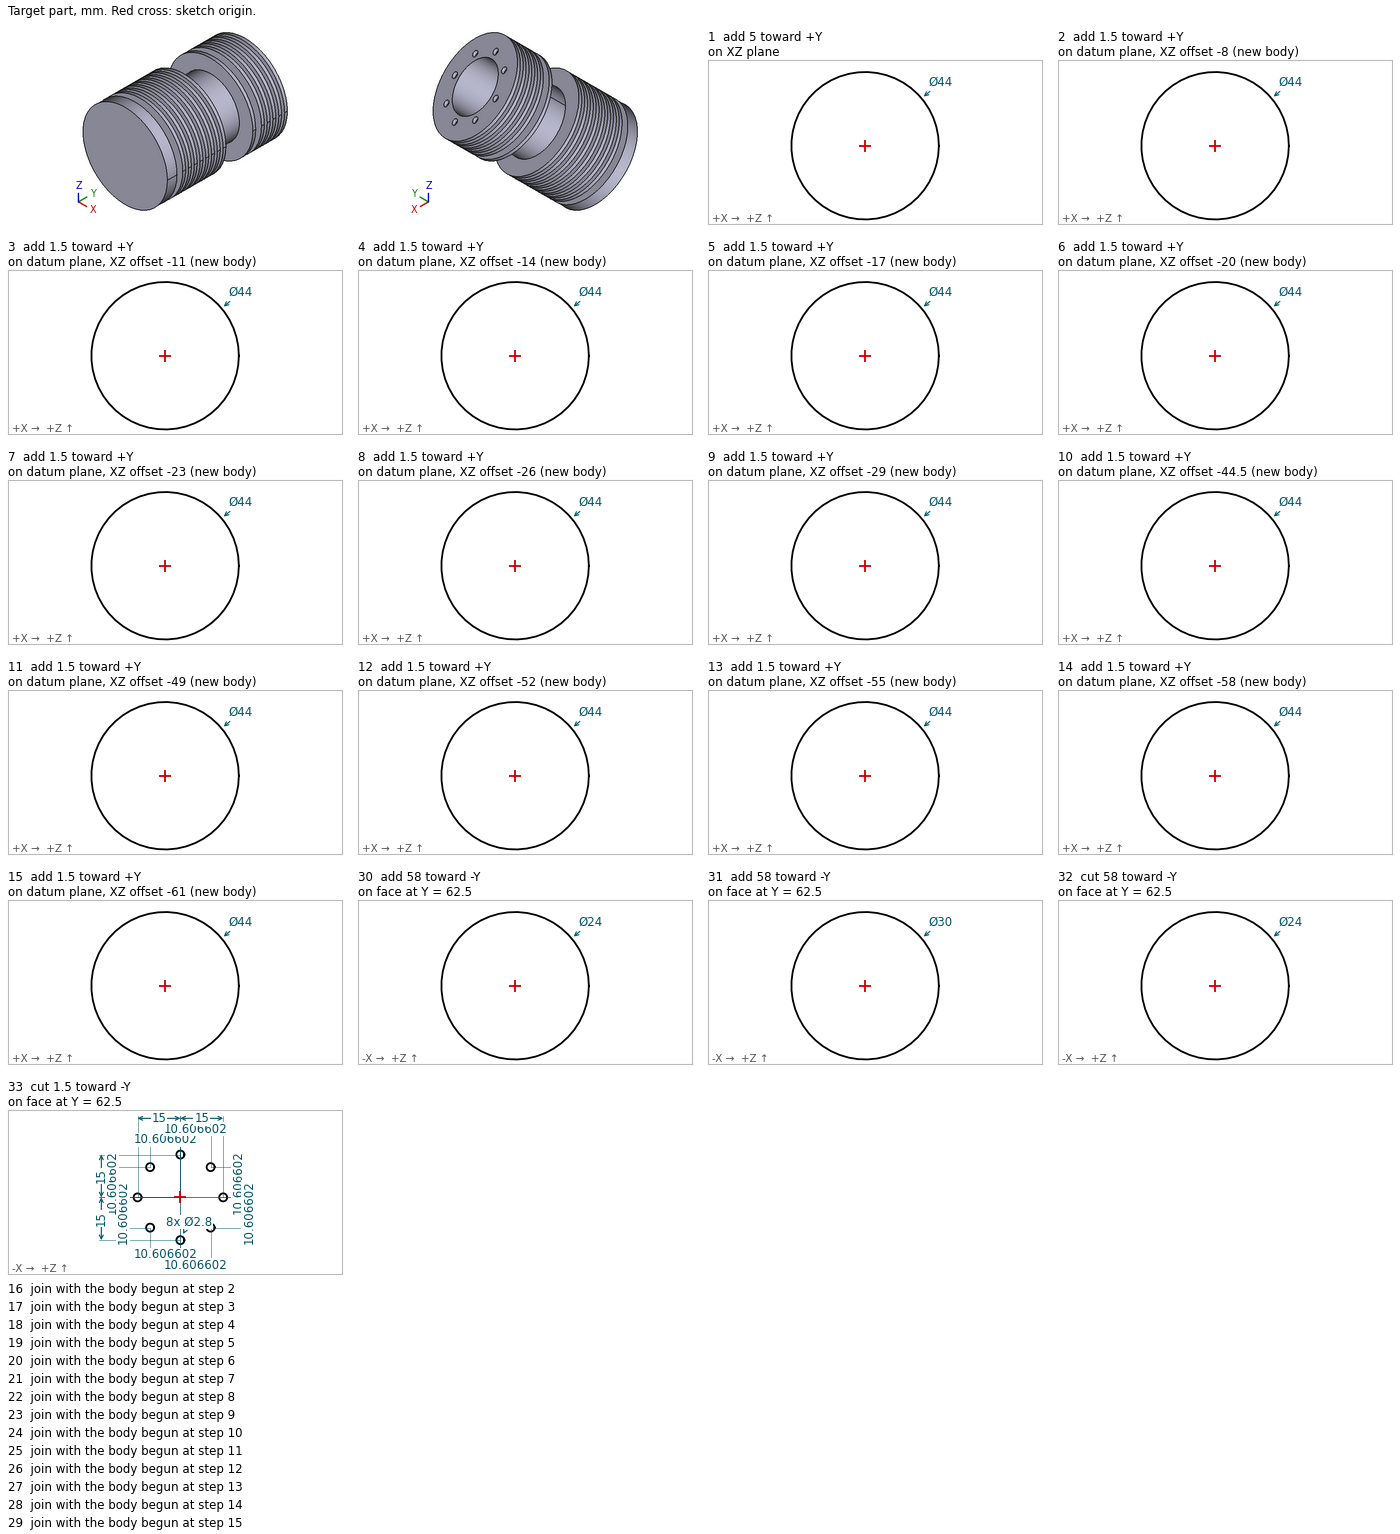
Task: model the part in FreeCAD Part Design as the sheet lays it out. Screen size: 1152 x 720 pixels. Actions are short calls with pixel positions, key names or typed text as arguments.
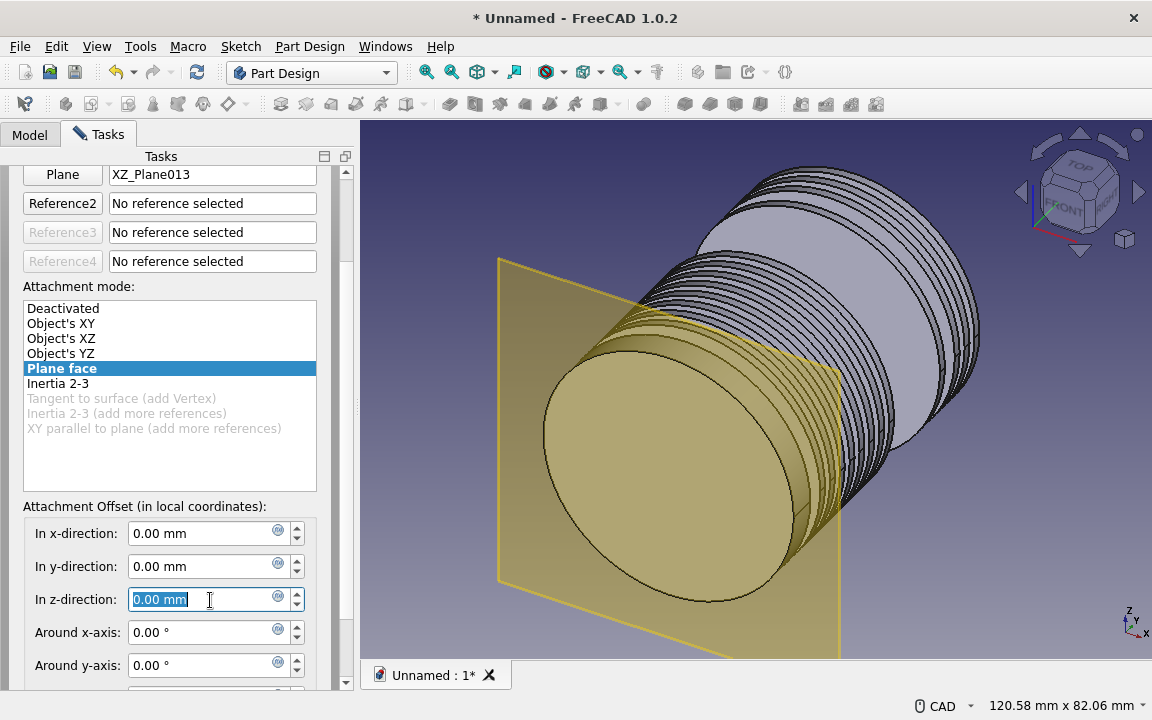
text(-58)
key(Tab)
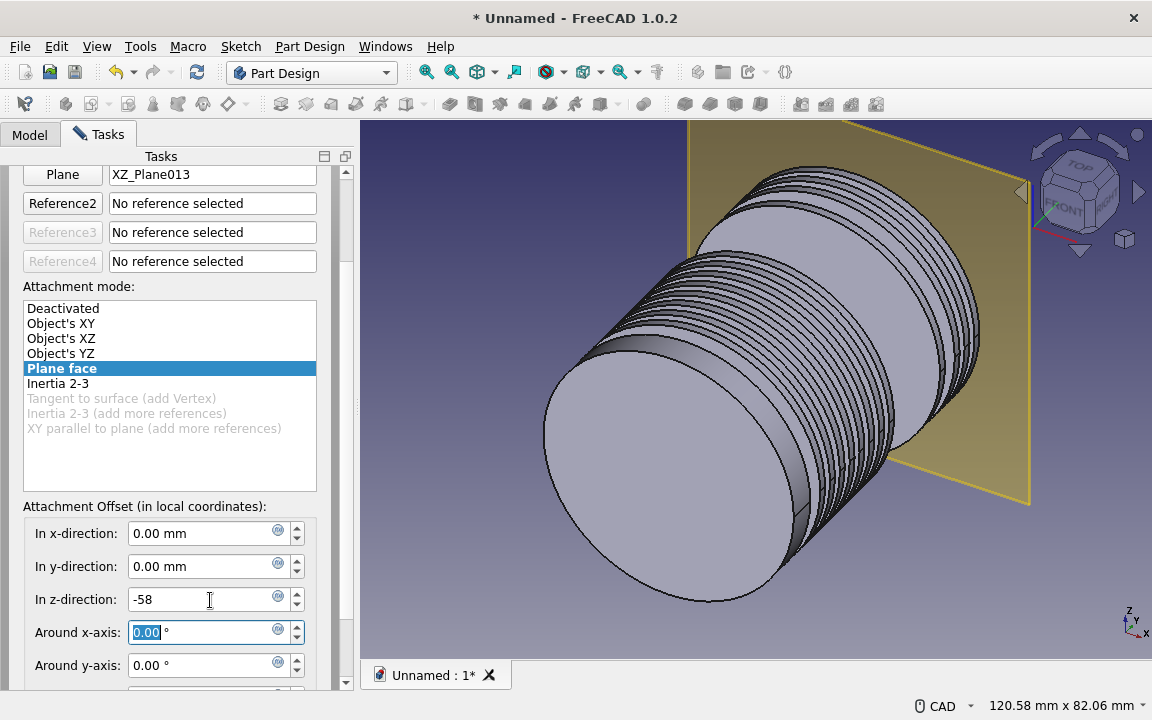
scroll(346, 428, up, 3)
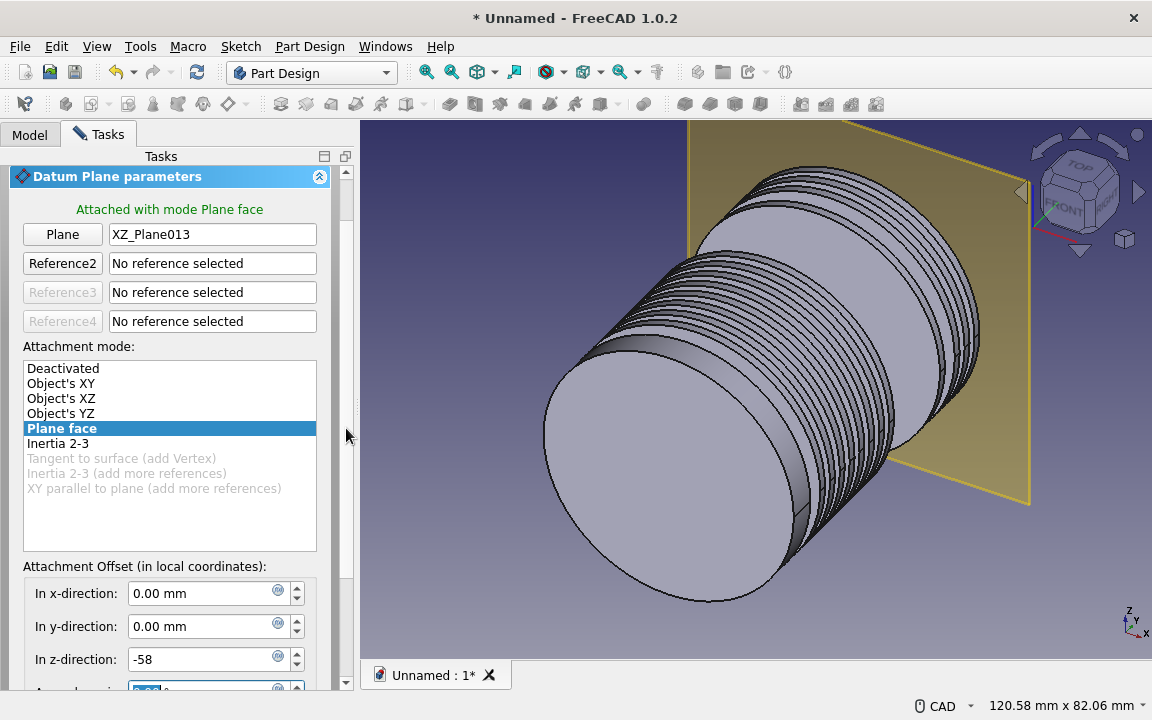
click(127, 195)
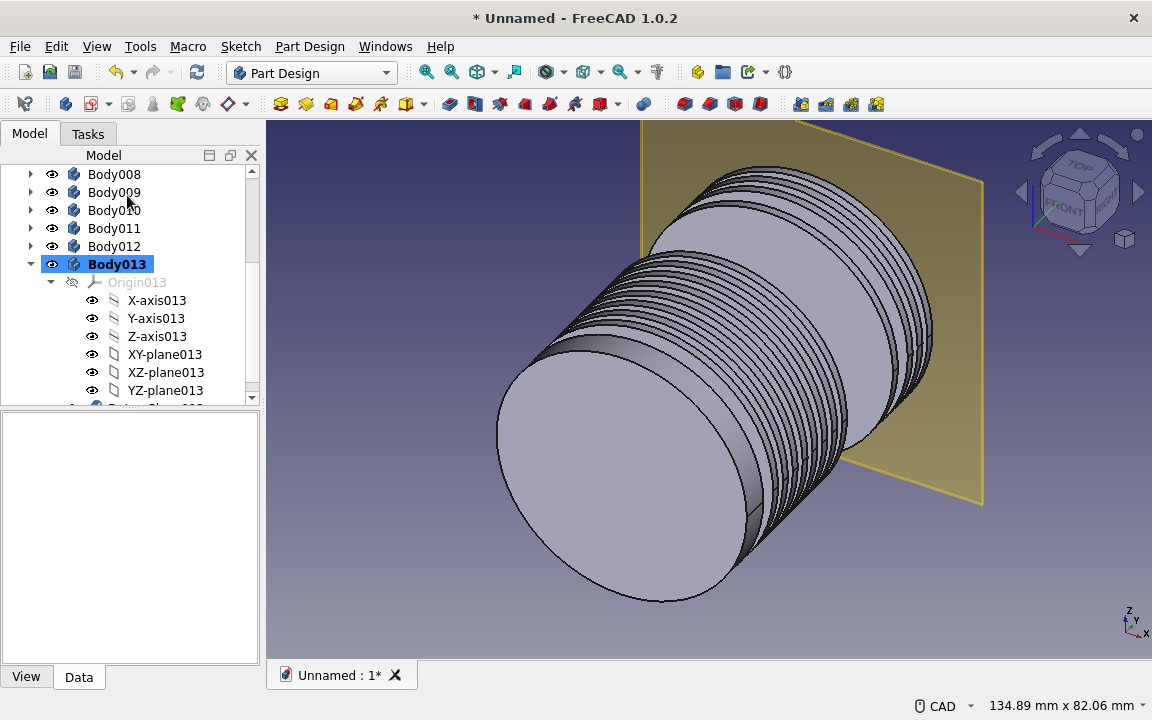
scroll(121, 278, down, 3)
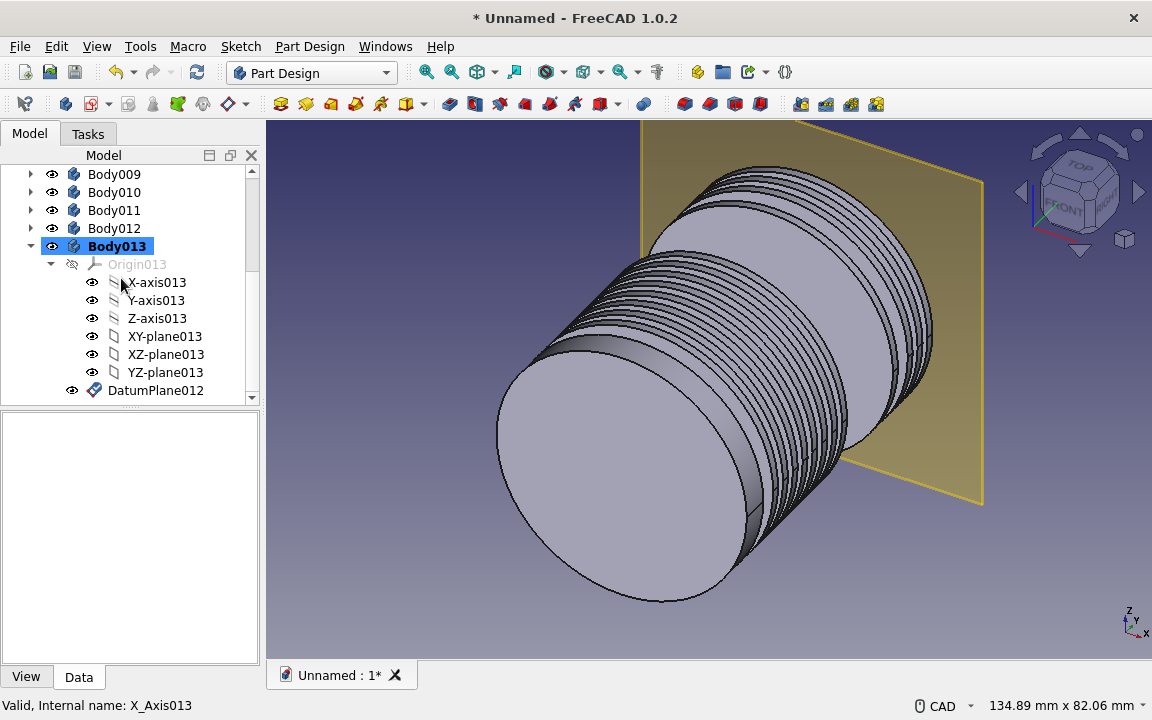
click(117, 390)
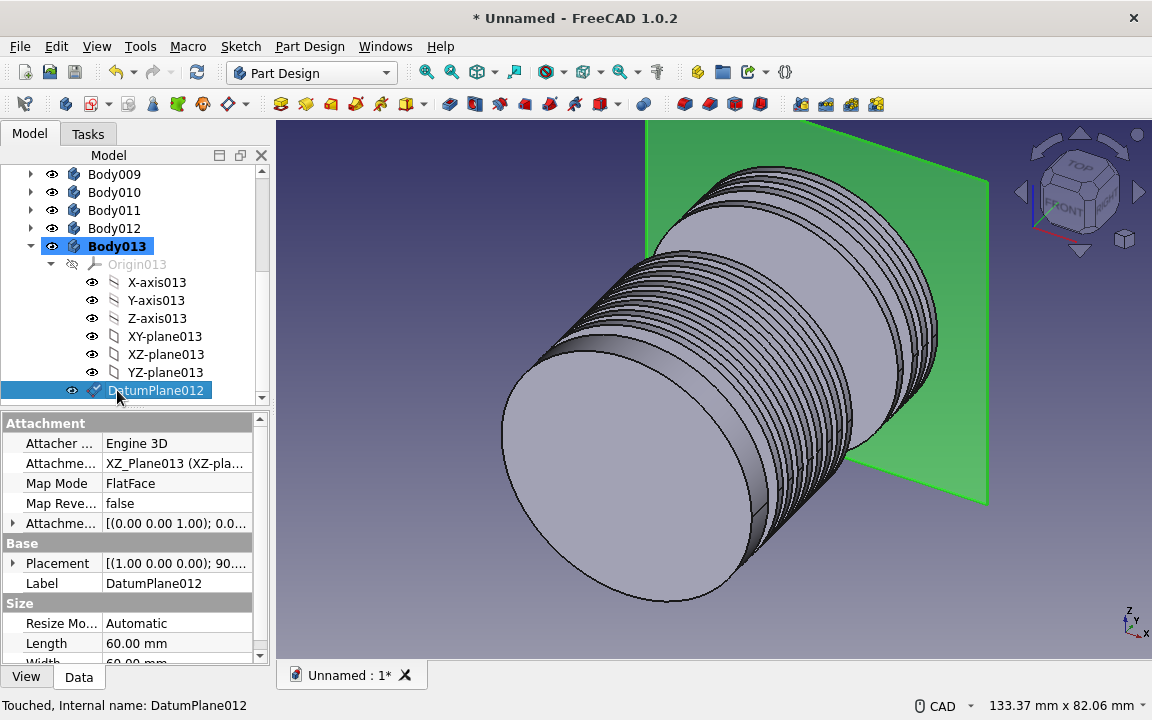
click(90, 104)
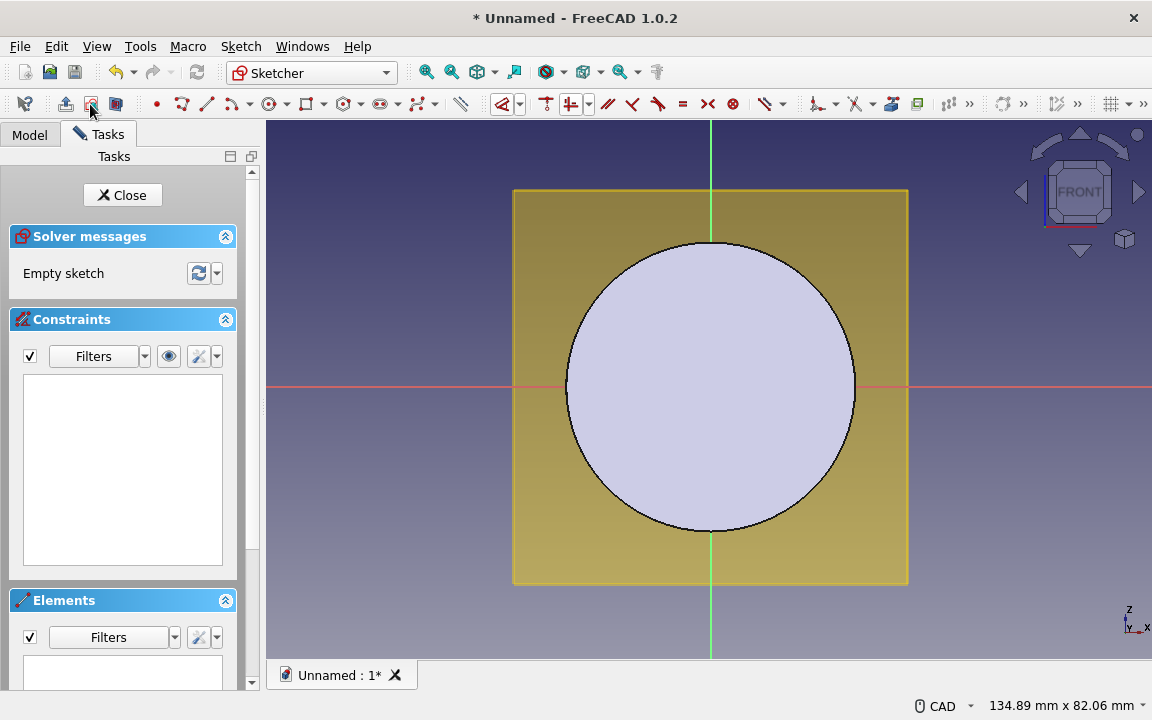
key(g)
key(c)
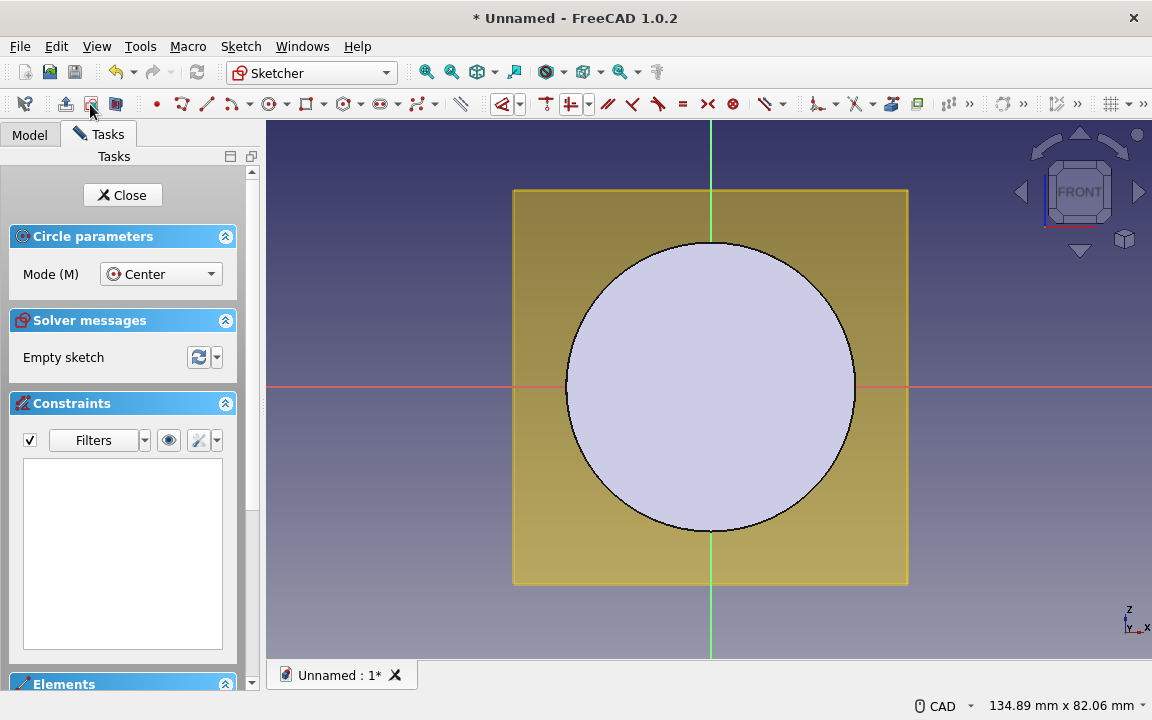
click(711, 387)
click(813, 285)
key(Escape)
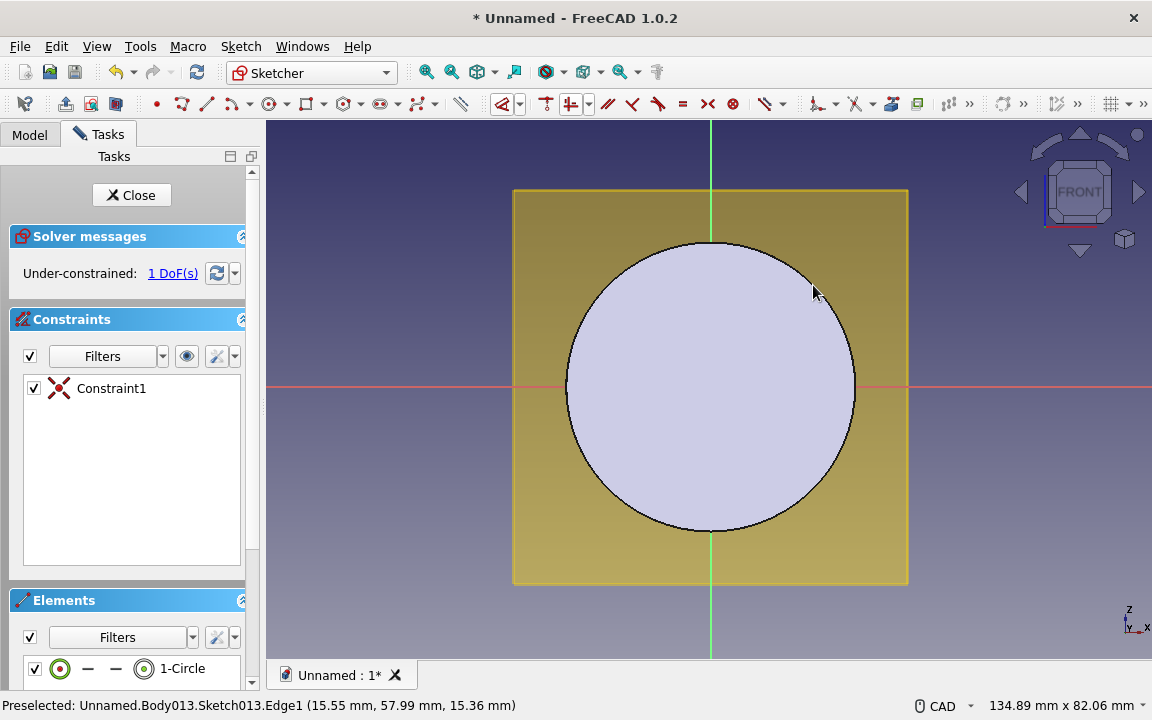
click(812, 285)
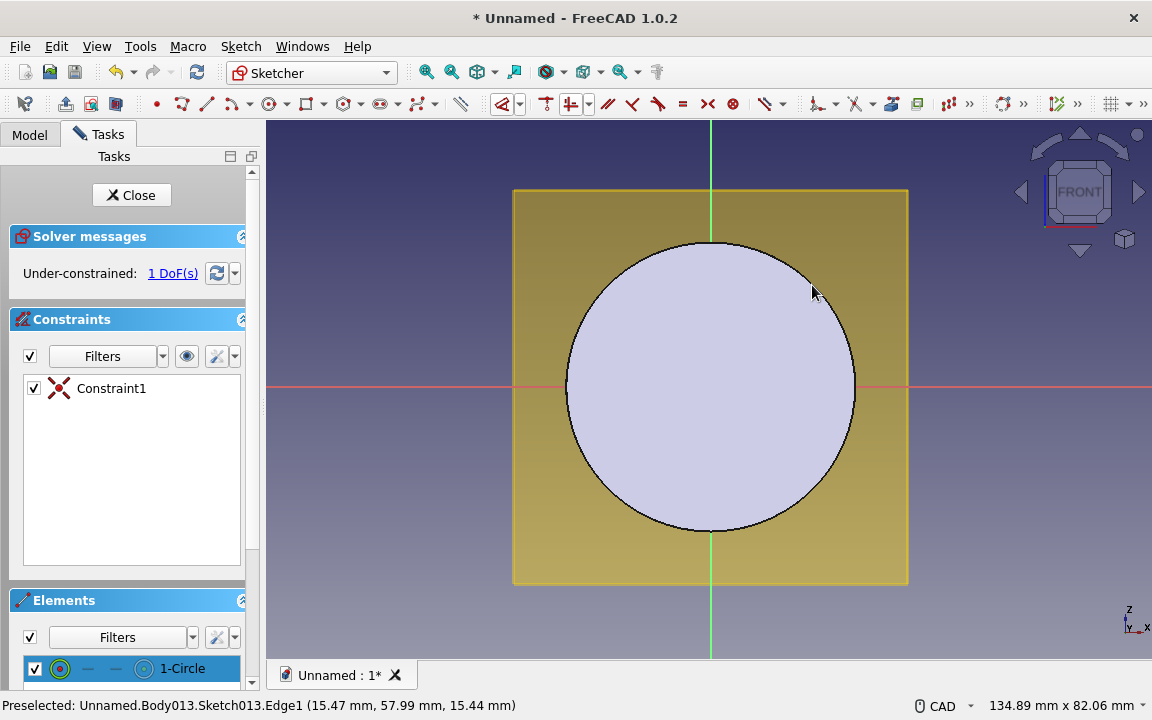
key(k)
key(o)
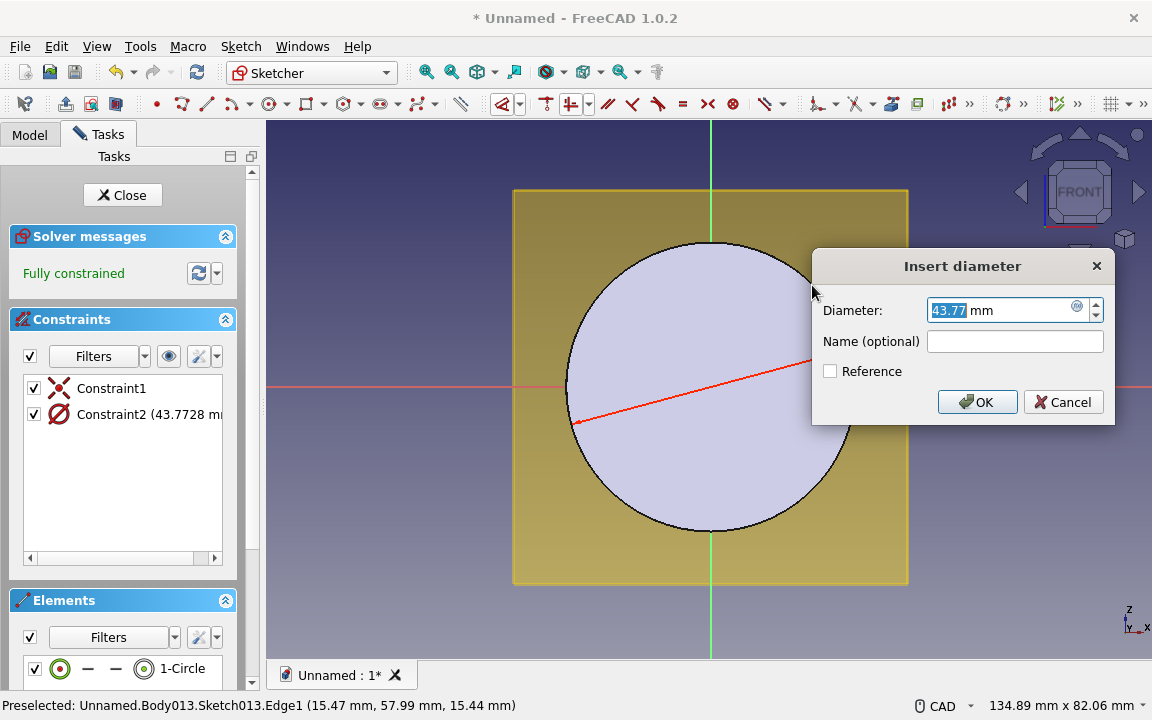
text(44)
key(Return)